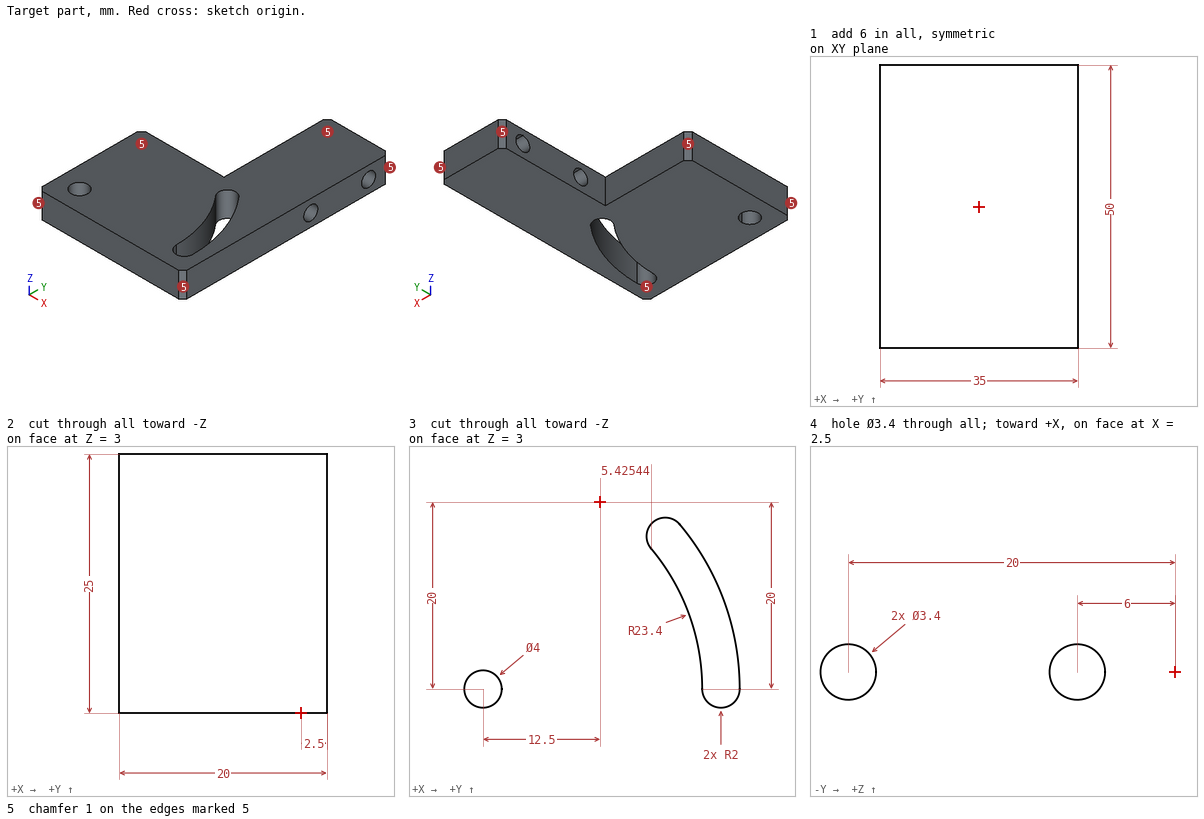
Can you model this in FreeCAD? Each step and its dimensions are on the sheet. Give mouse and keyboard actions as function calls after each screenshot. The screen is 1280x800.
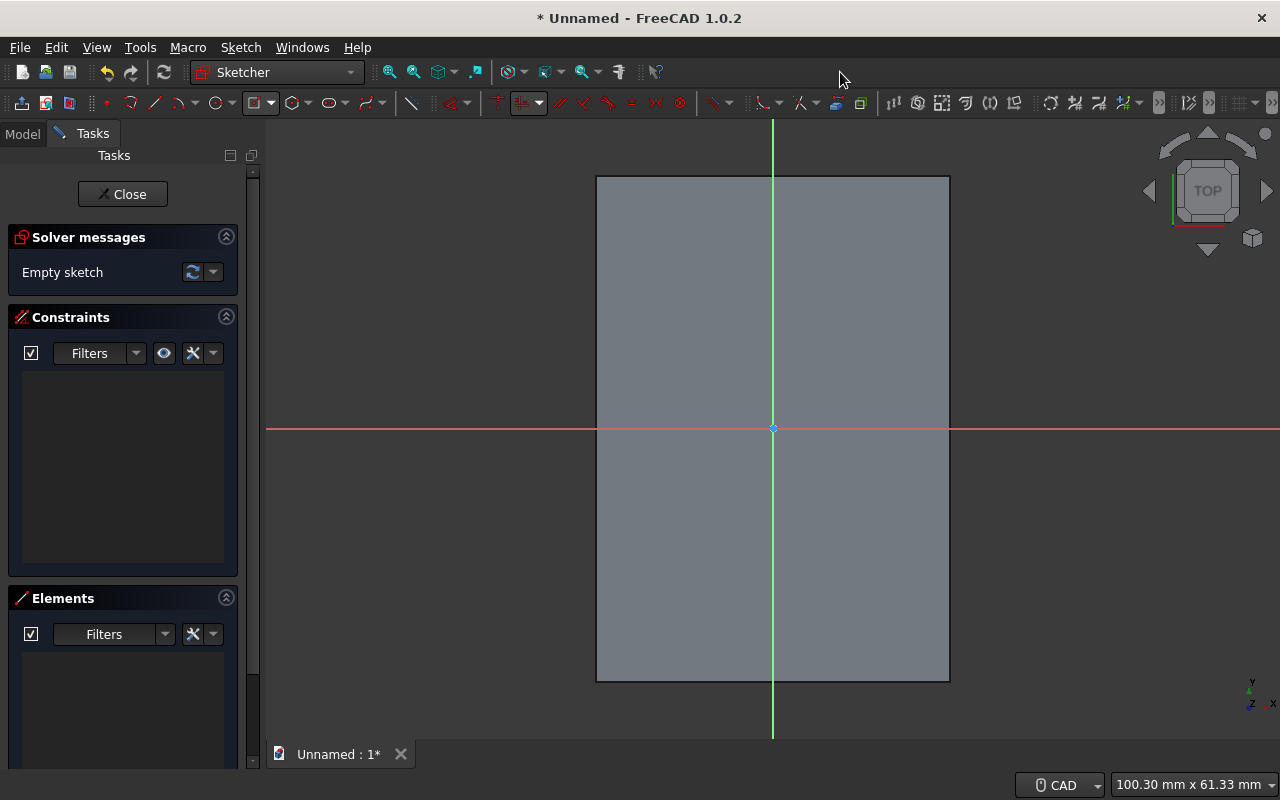
scroll(682, 147, up, 2)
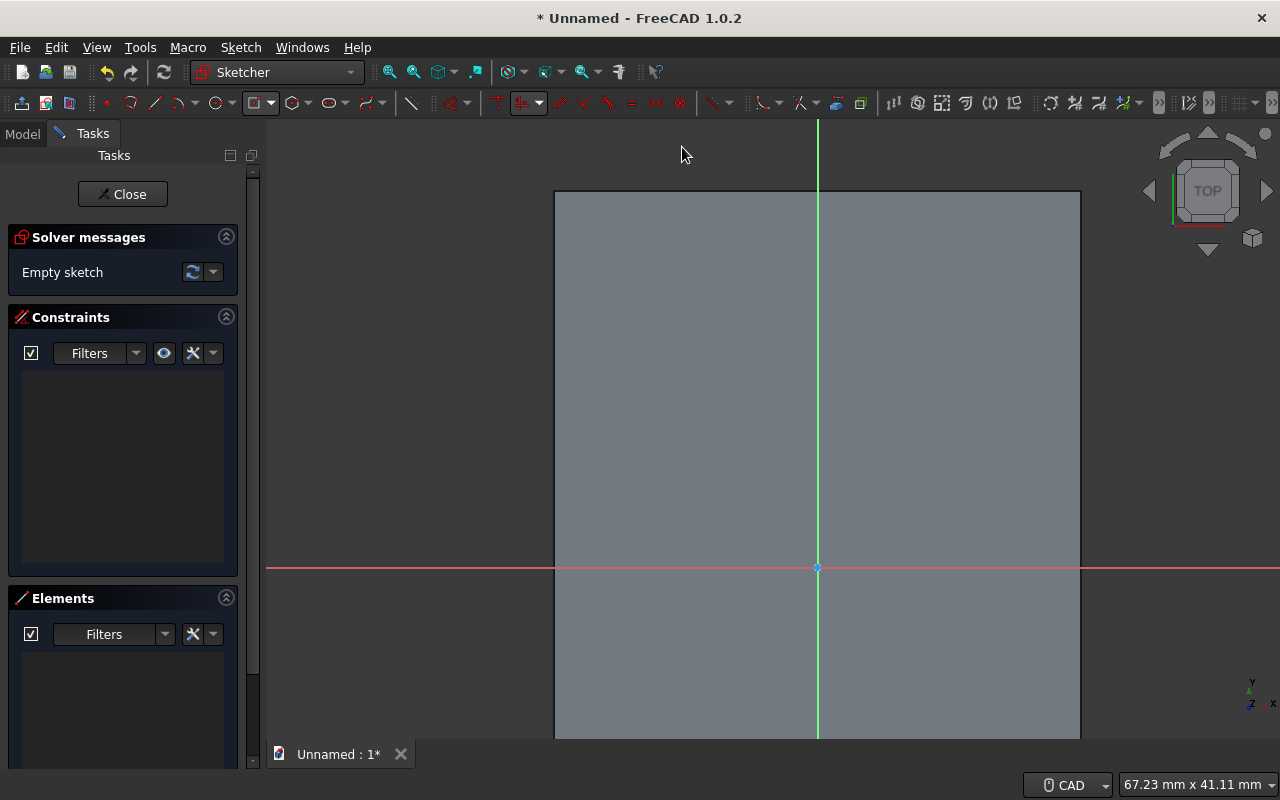
key(g)
key(r)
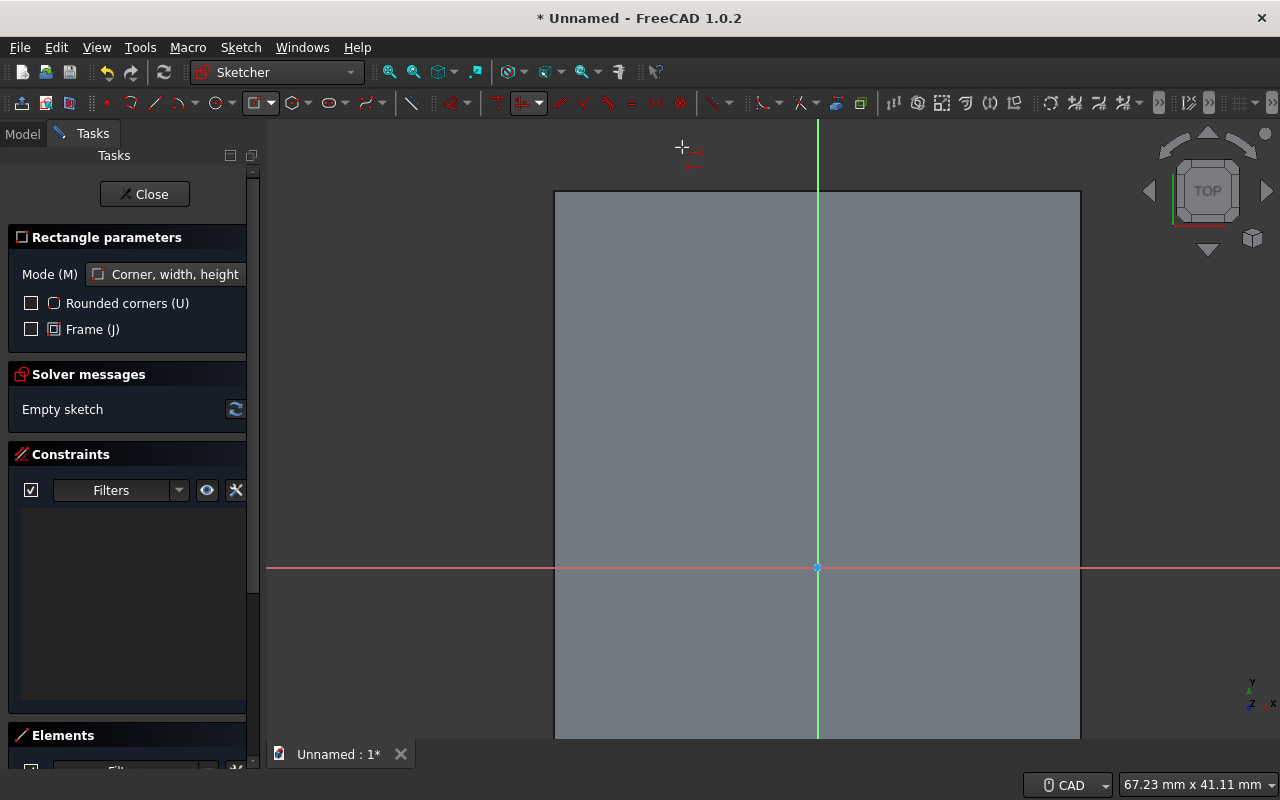
click(554, 191)
click(855, 568)
key(Escape)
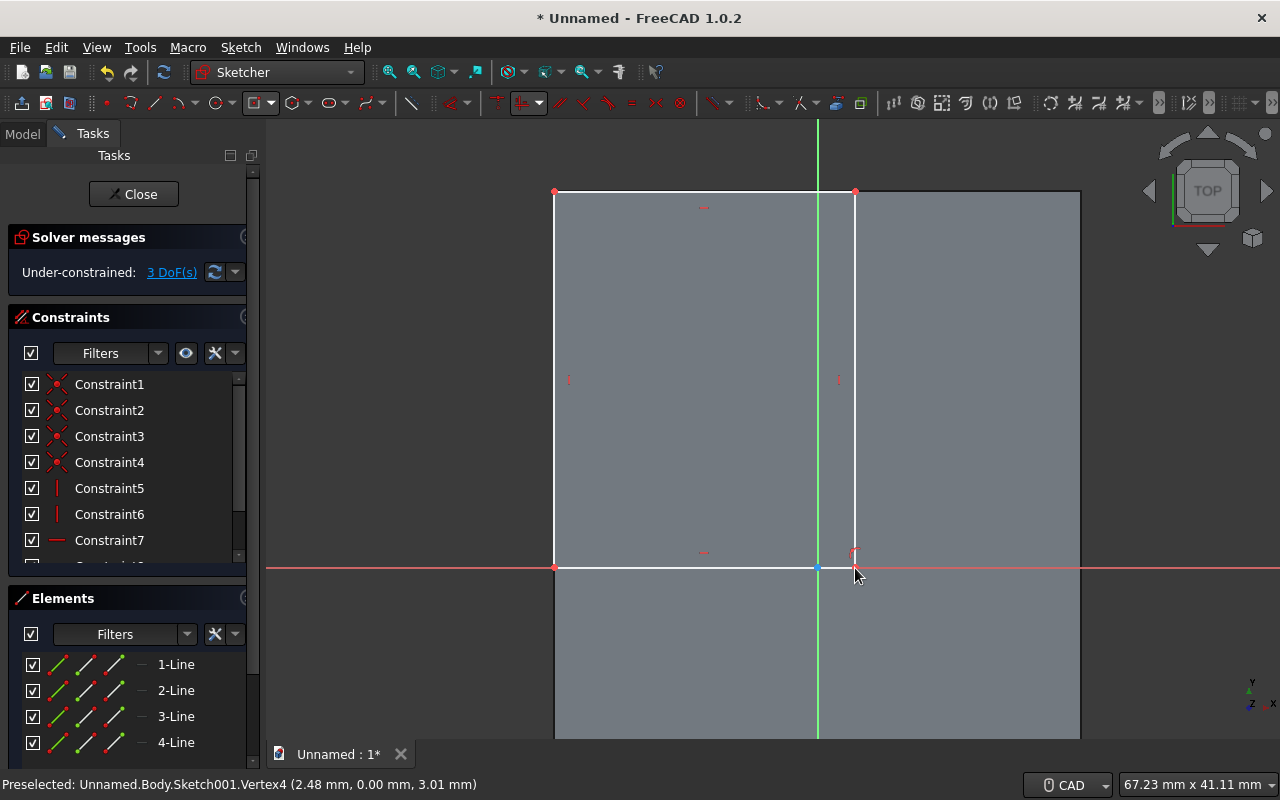
click(450, 104)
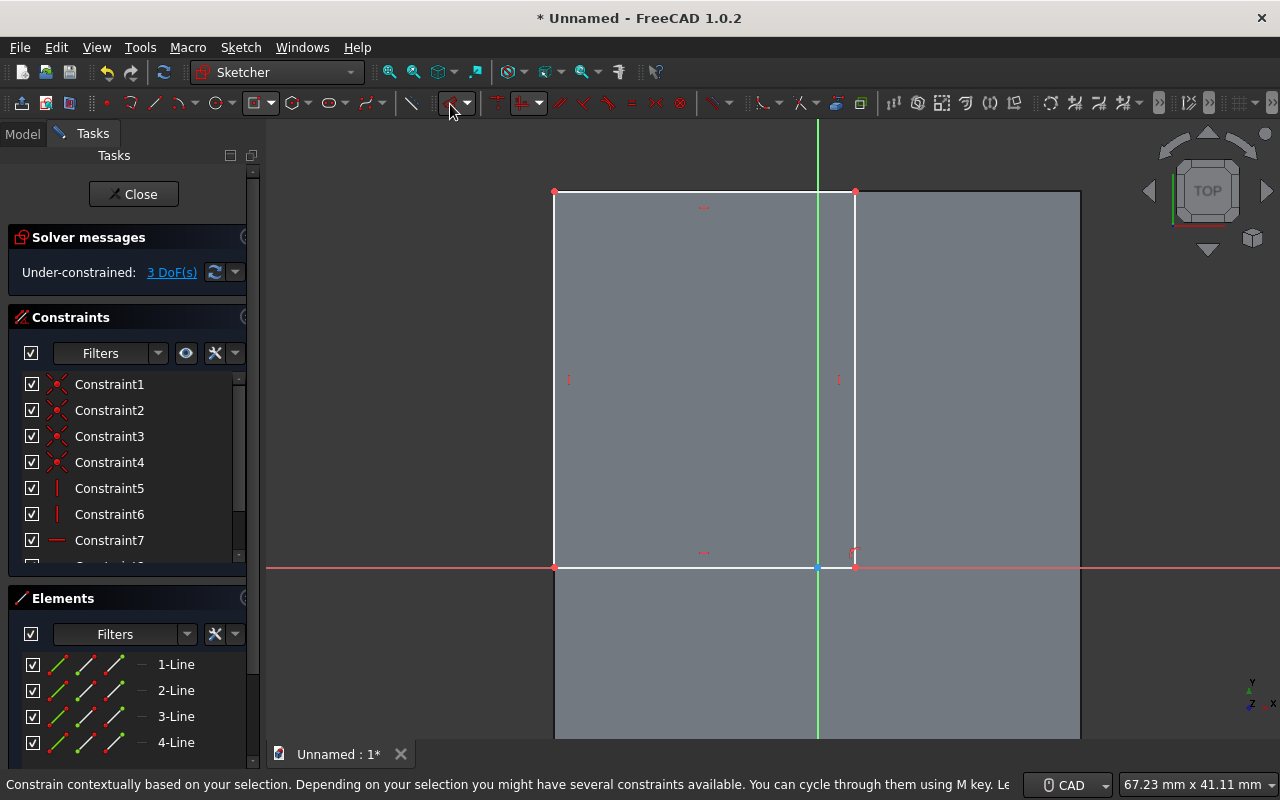
click(554, 305)
click(520, 380)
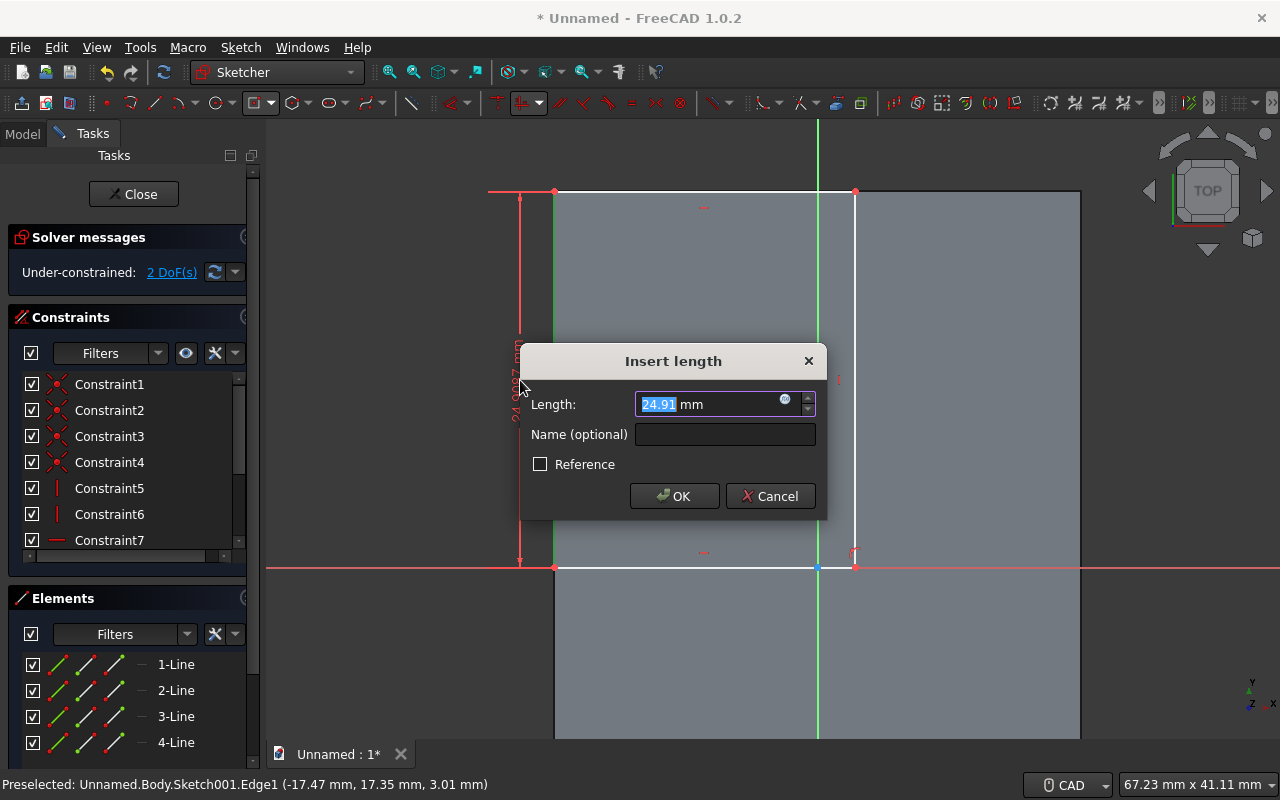
text(25)
key(Return)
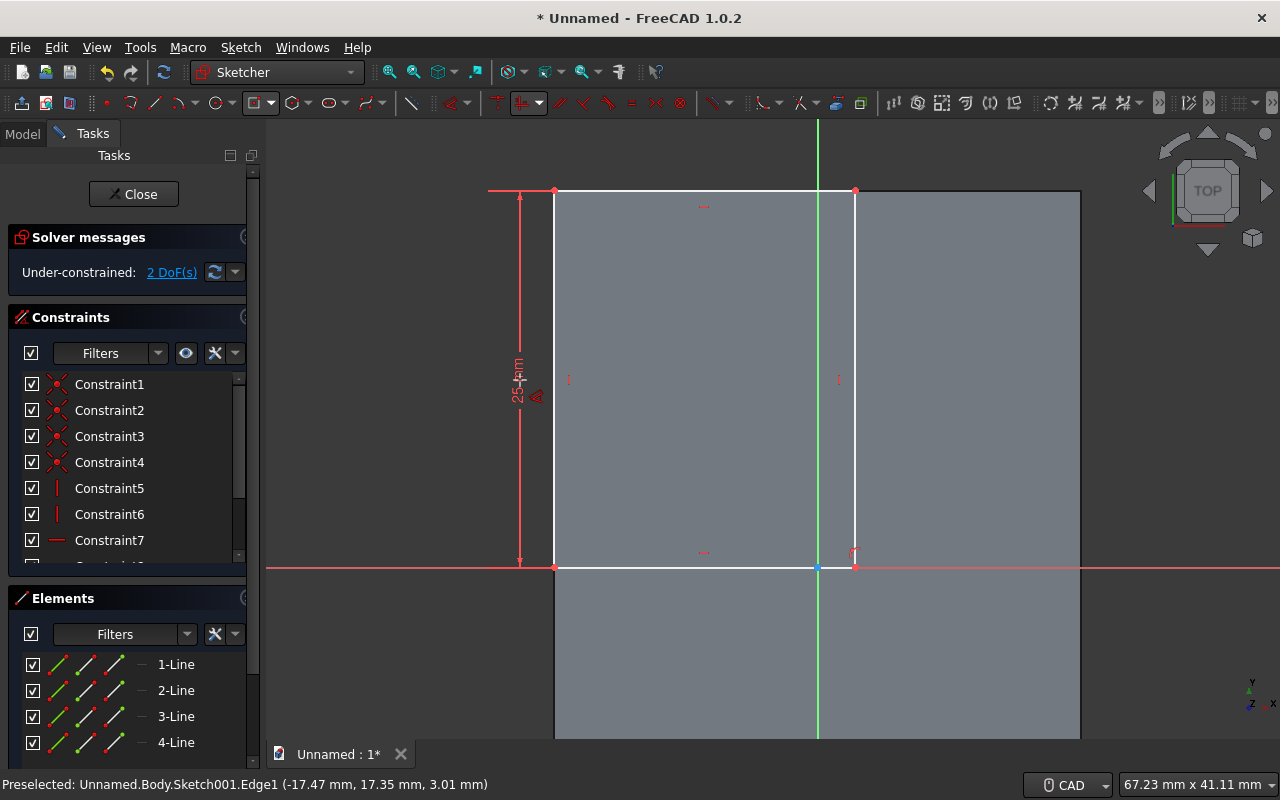
click(644, 568)
click(704, 602)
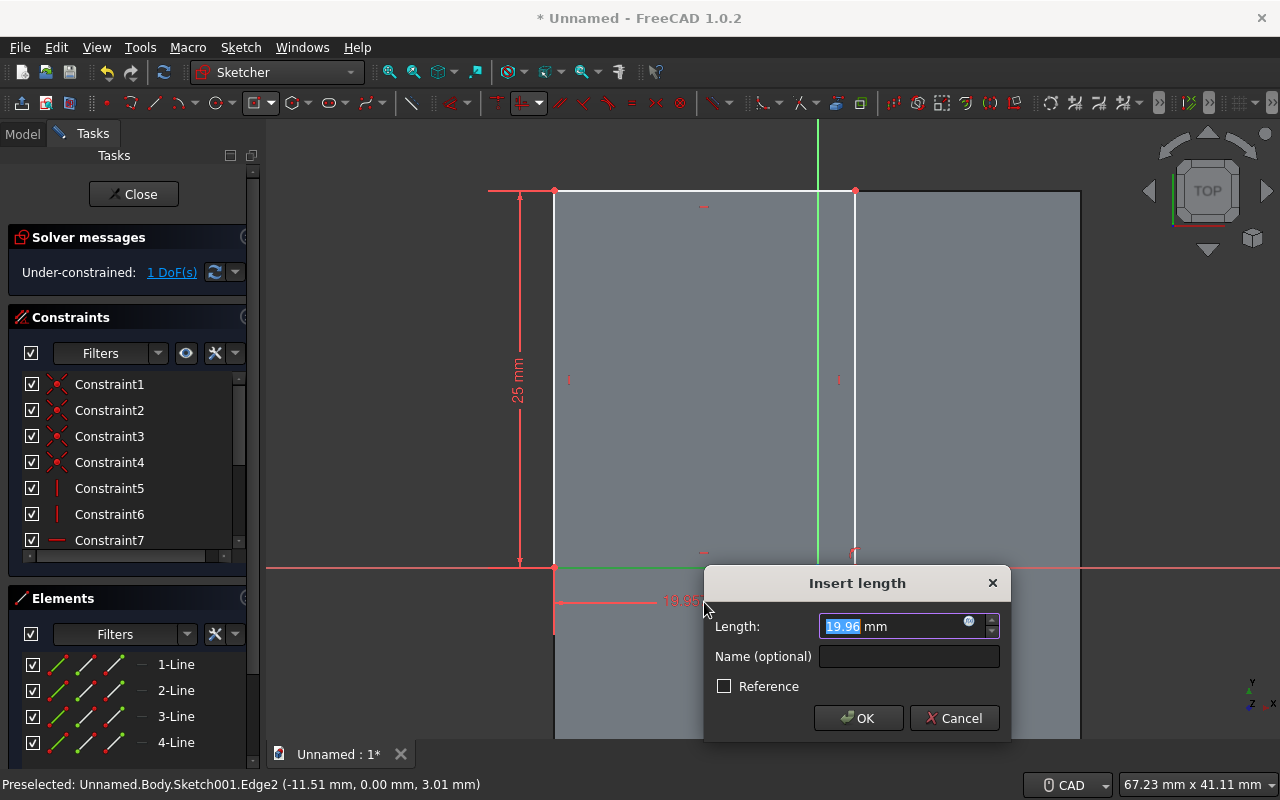
text(20)
key(Return)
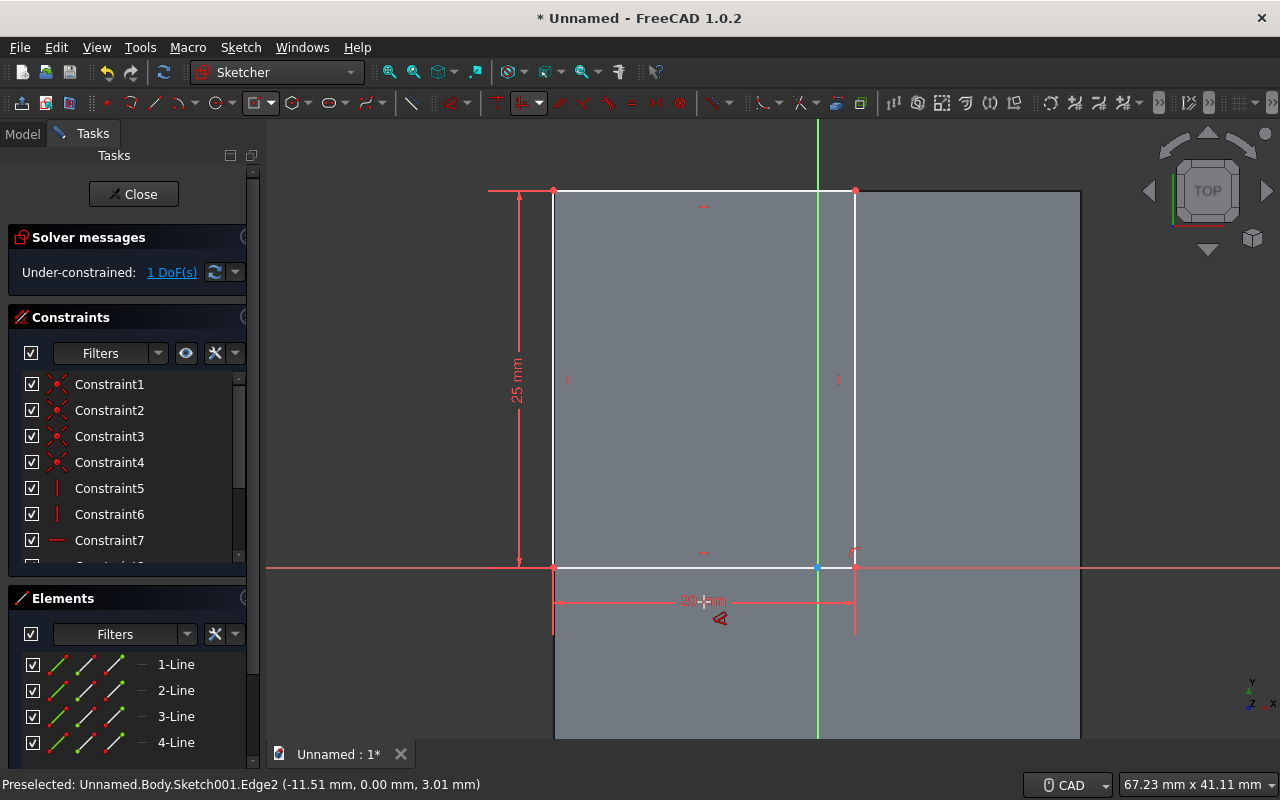
click(855, 568)
click(836, 602)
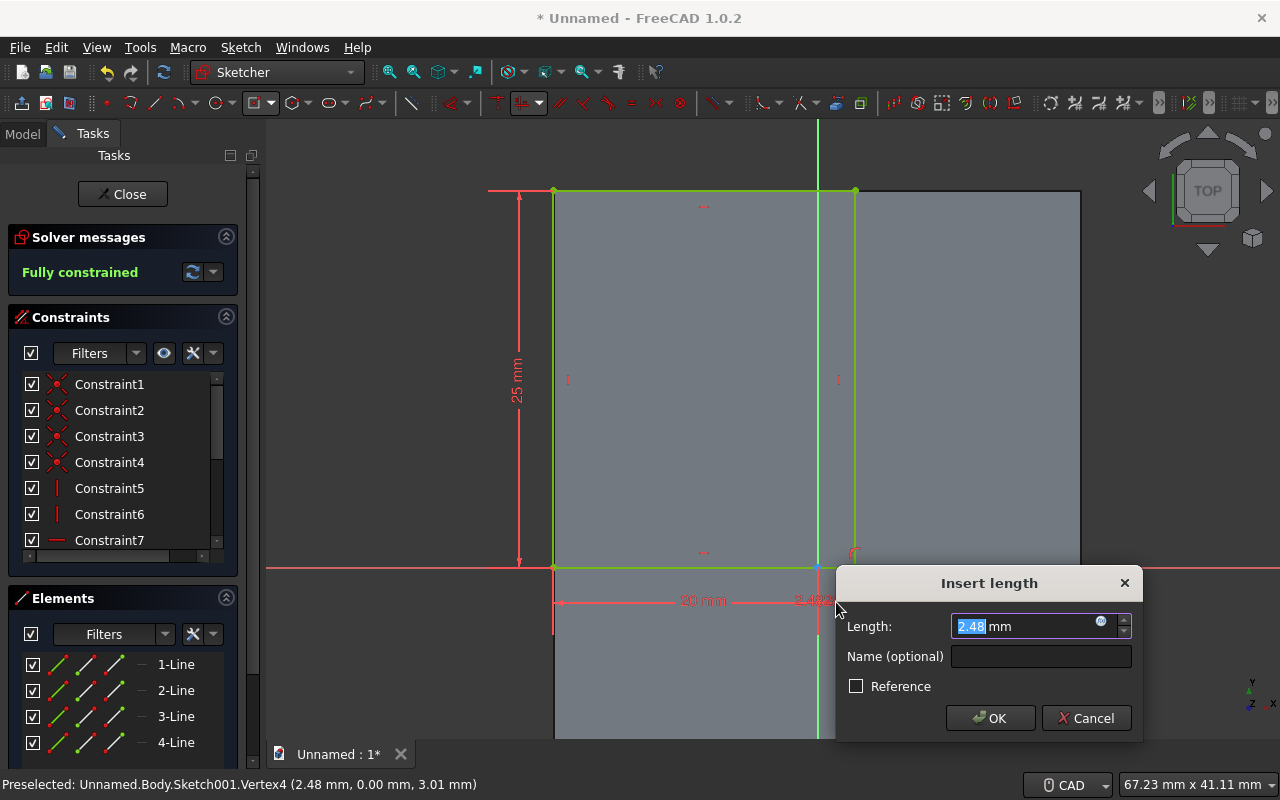
text(2.5)
key(Return)
key(Escape)